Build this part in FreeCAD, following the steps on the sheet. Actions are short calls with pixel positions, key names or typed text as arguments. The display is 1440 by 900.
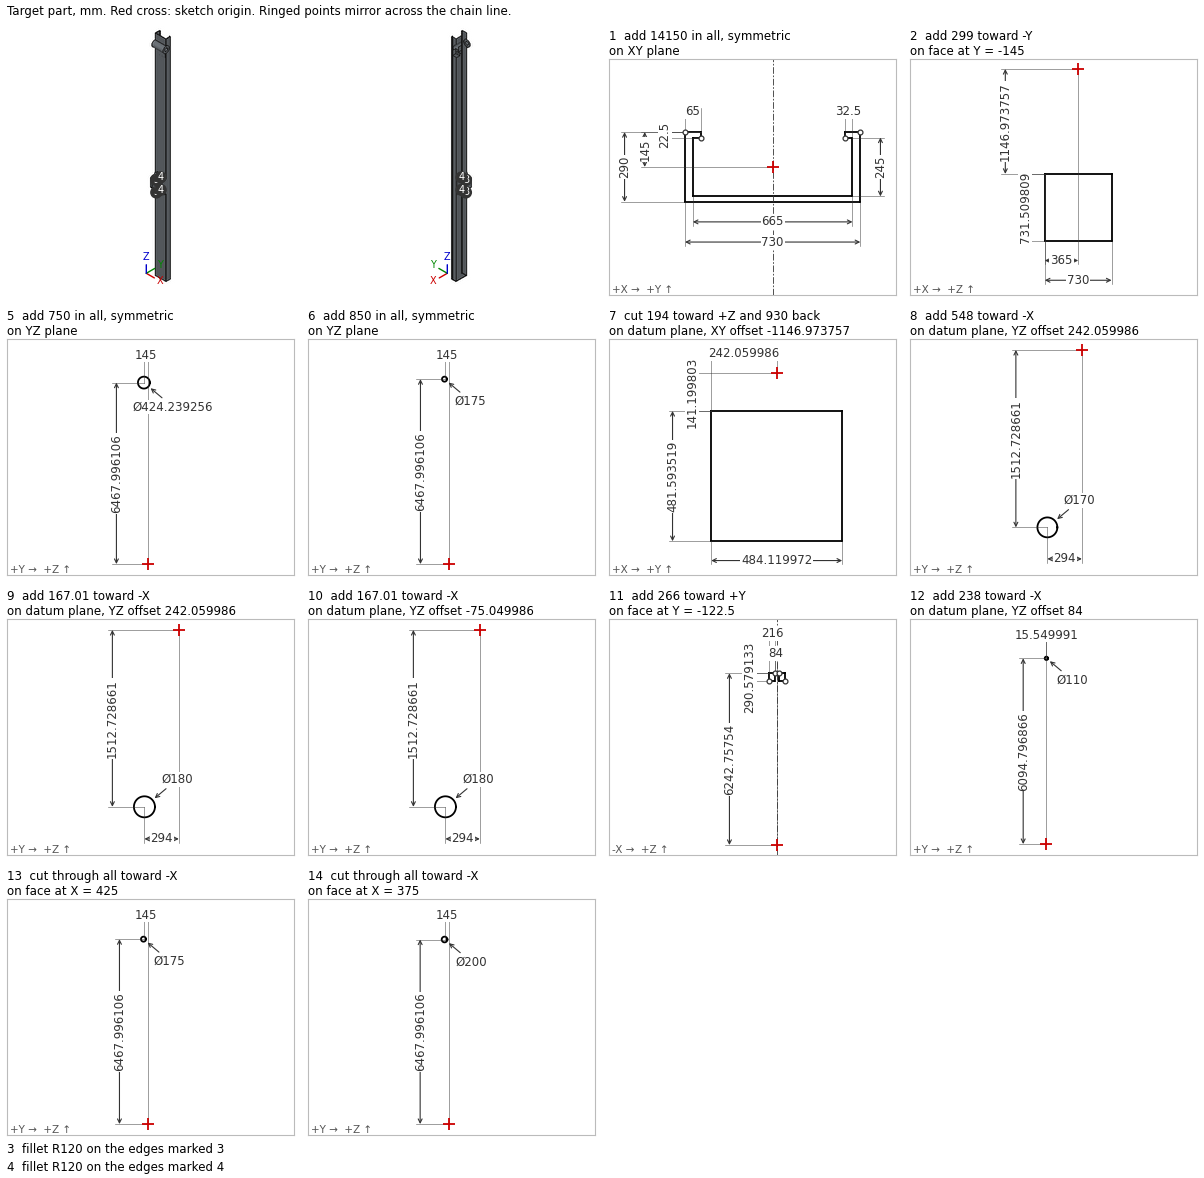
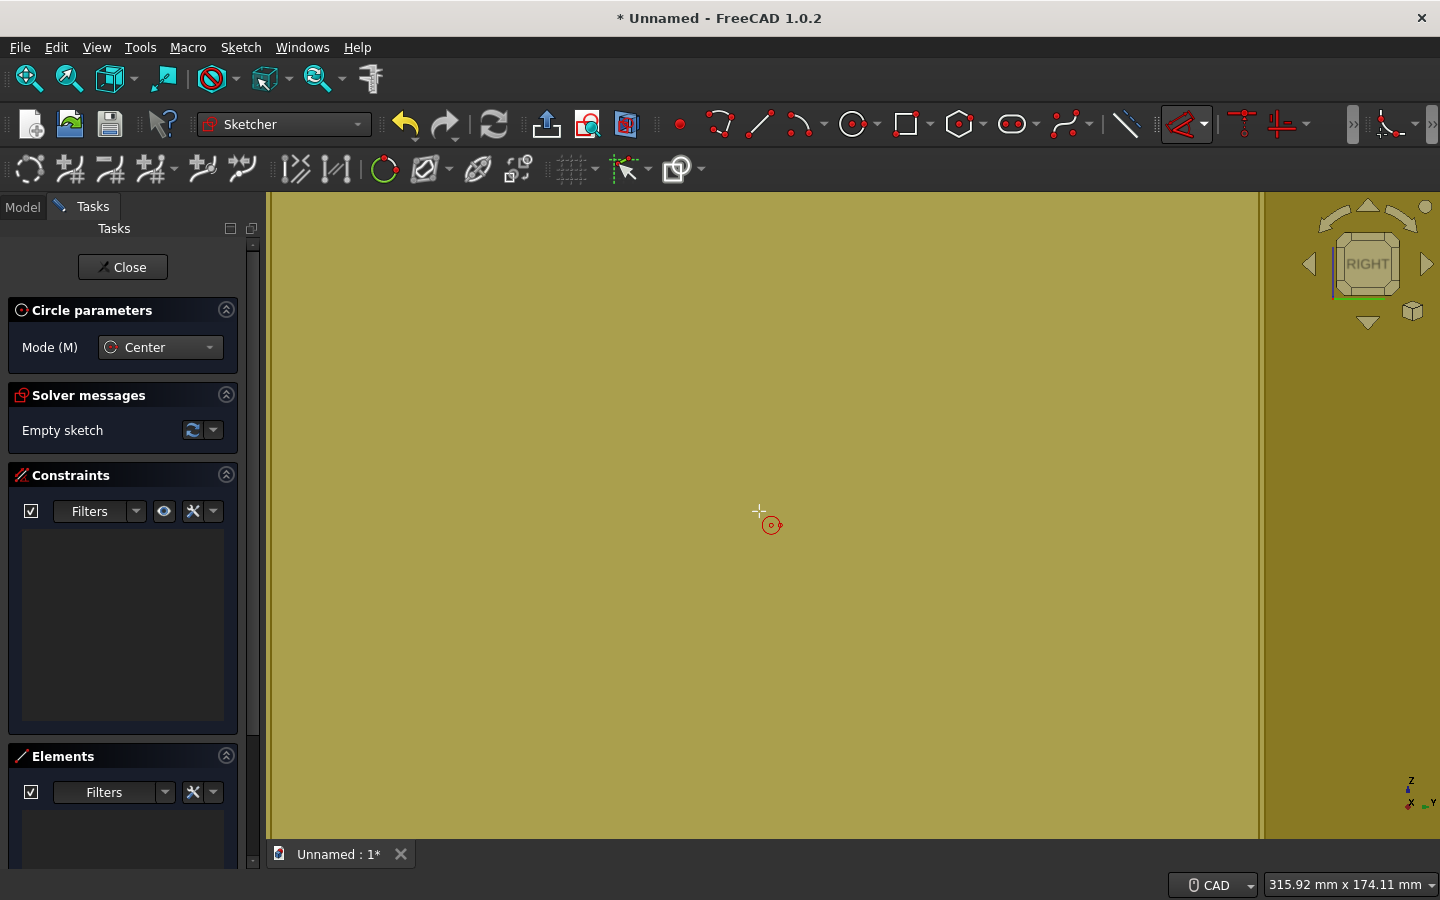
click(784, 513)
click(929, 369)
key(Escape)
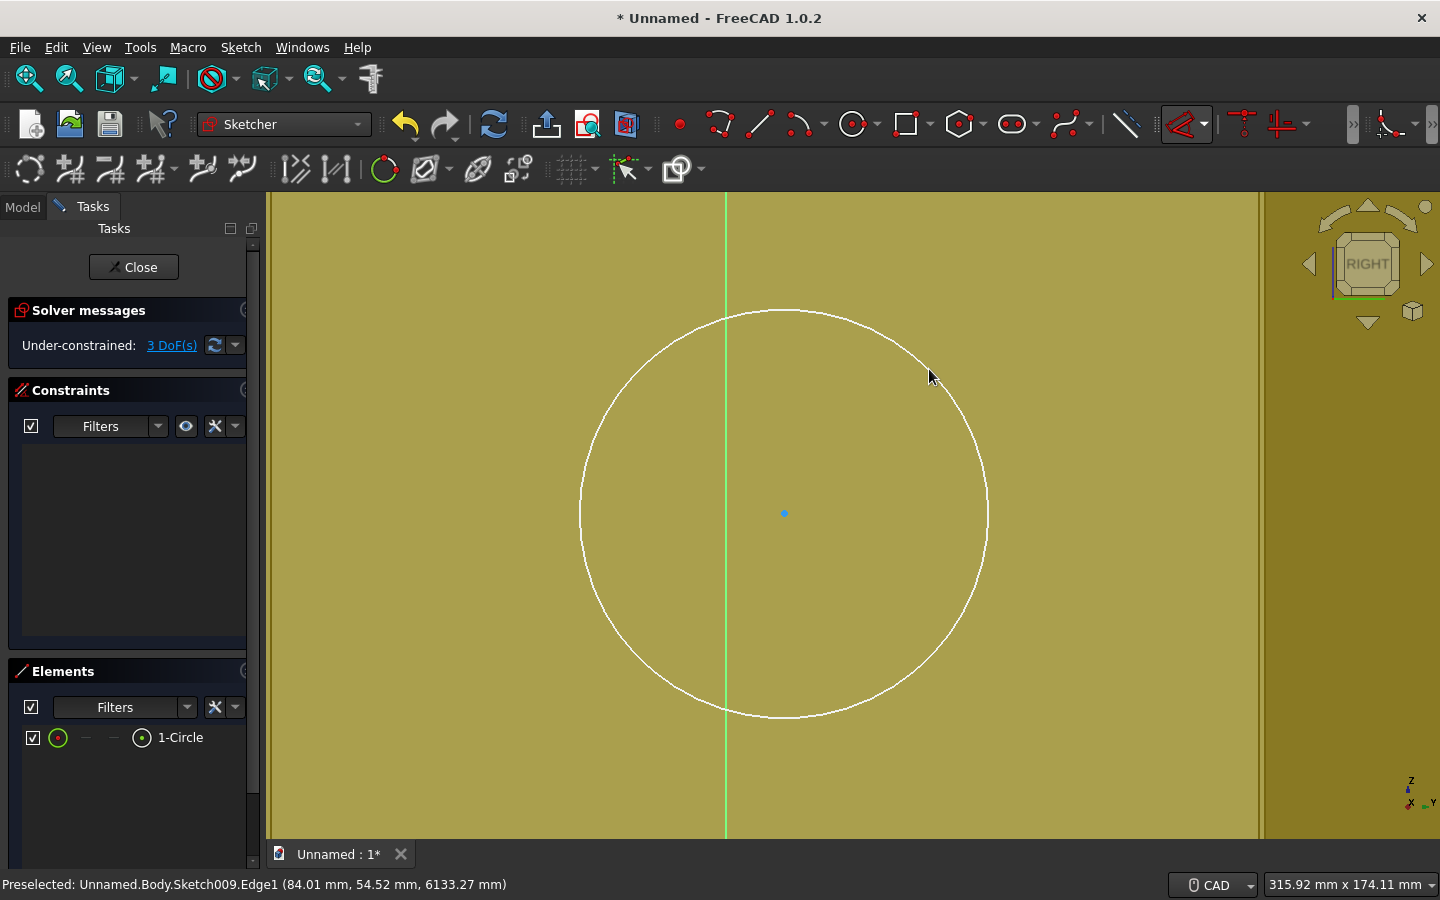
click(928, 369)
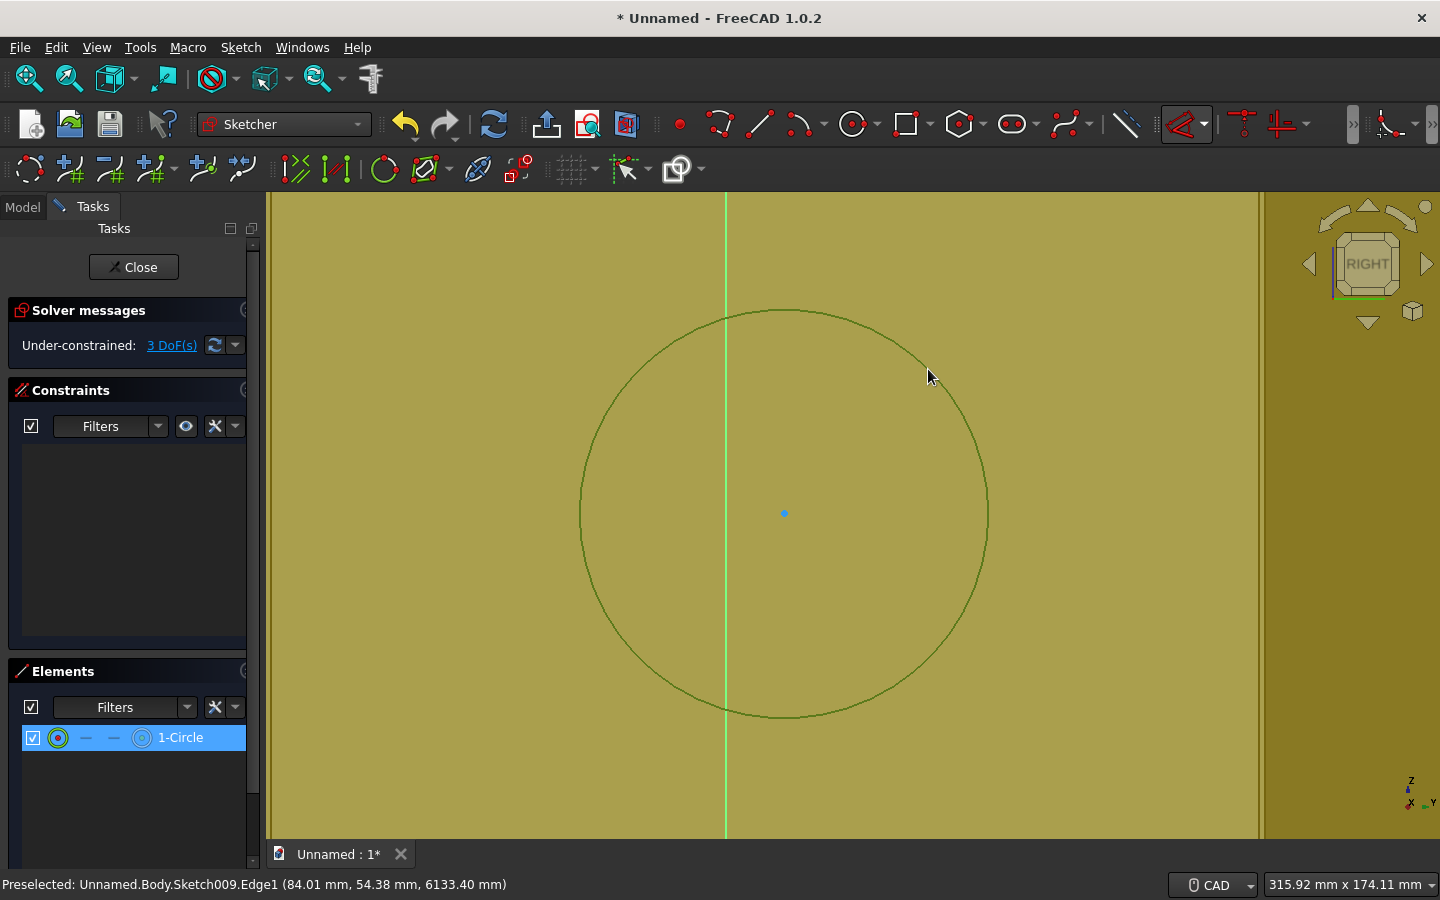
key(k)
key(o)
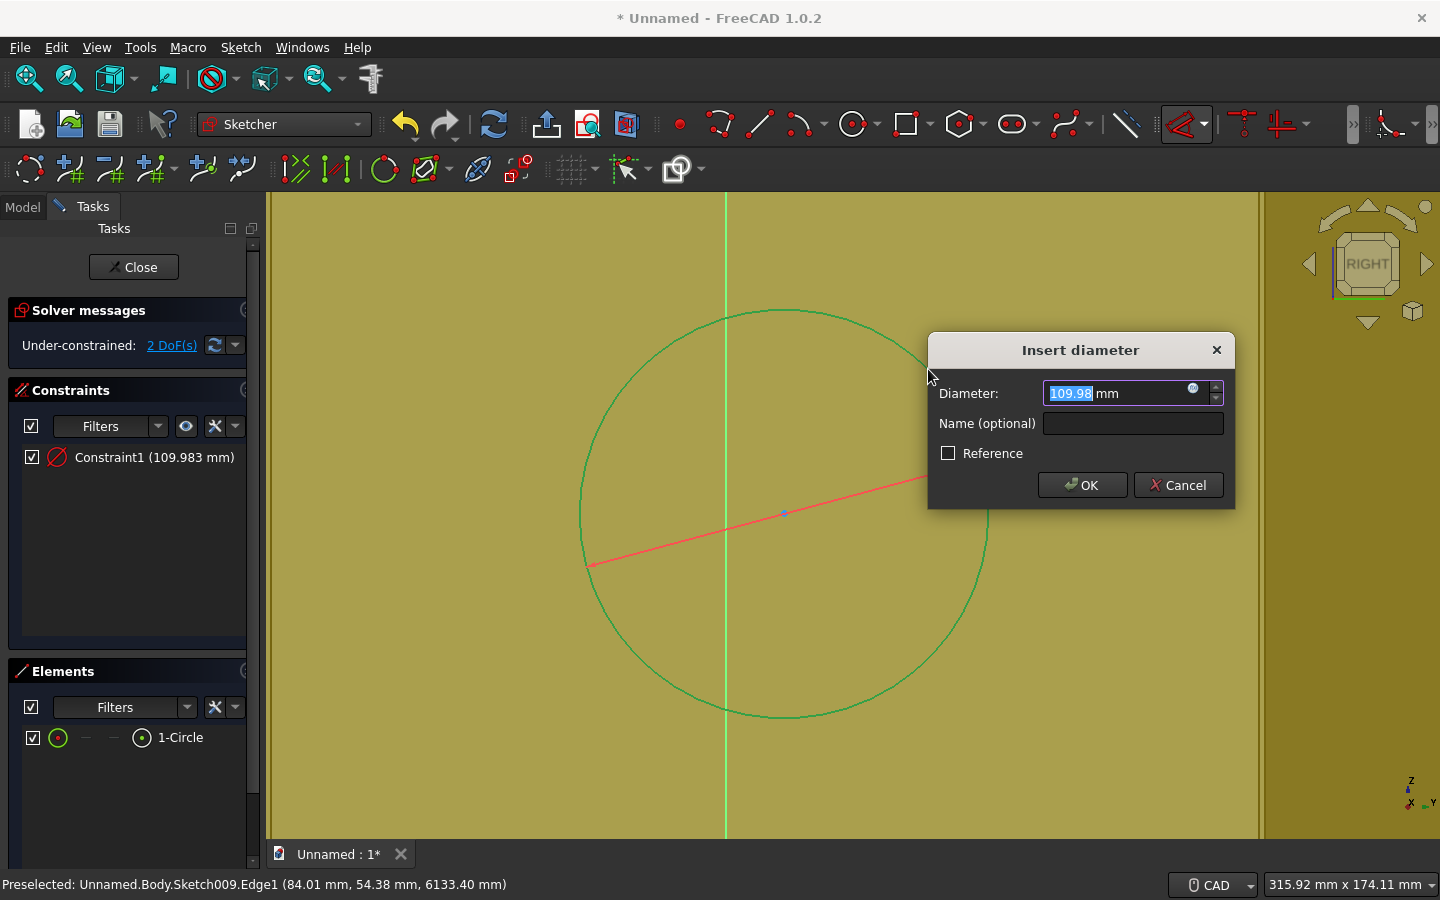
text(110)
key(Return)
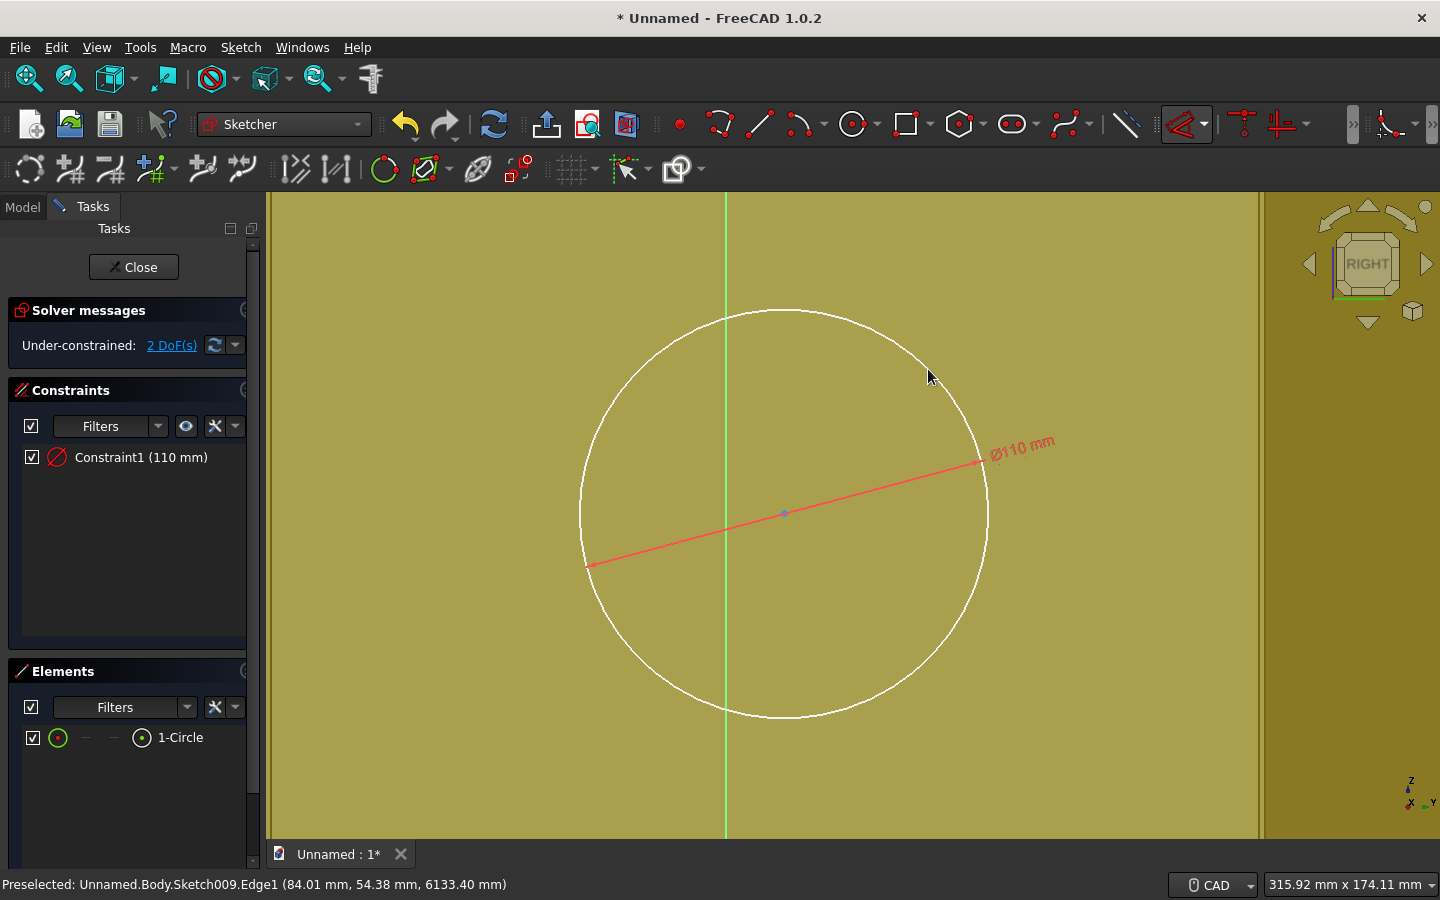
click(784, 514)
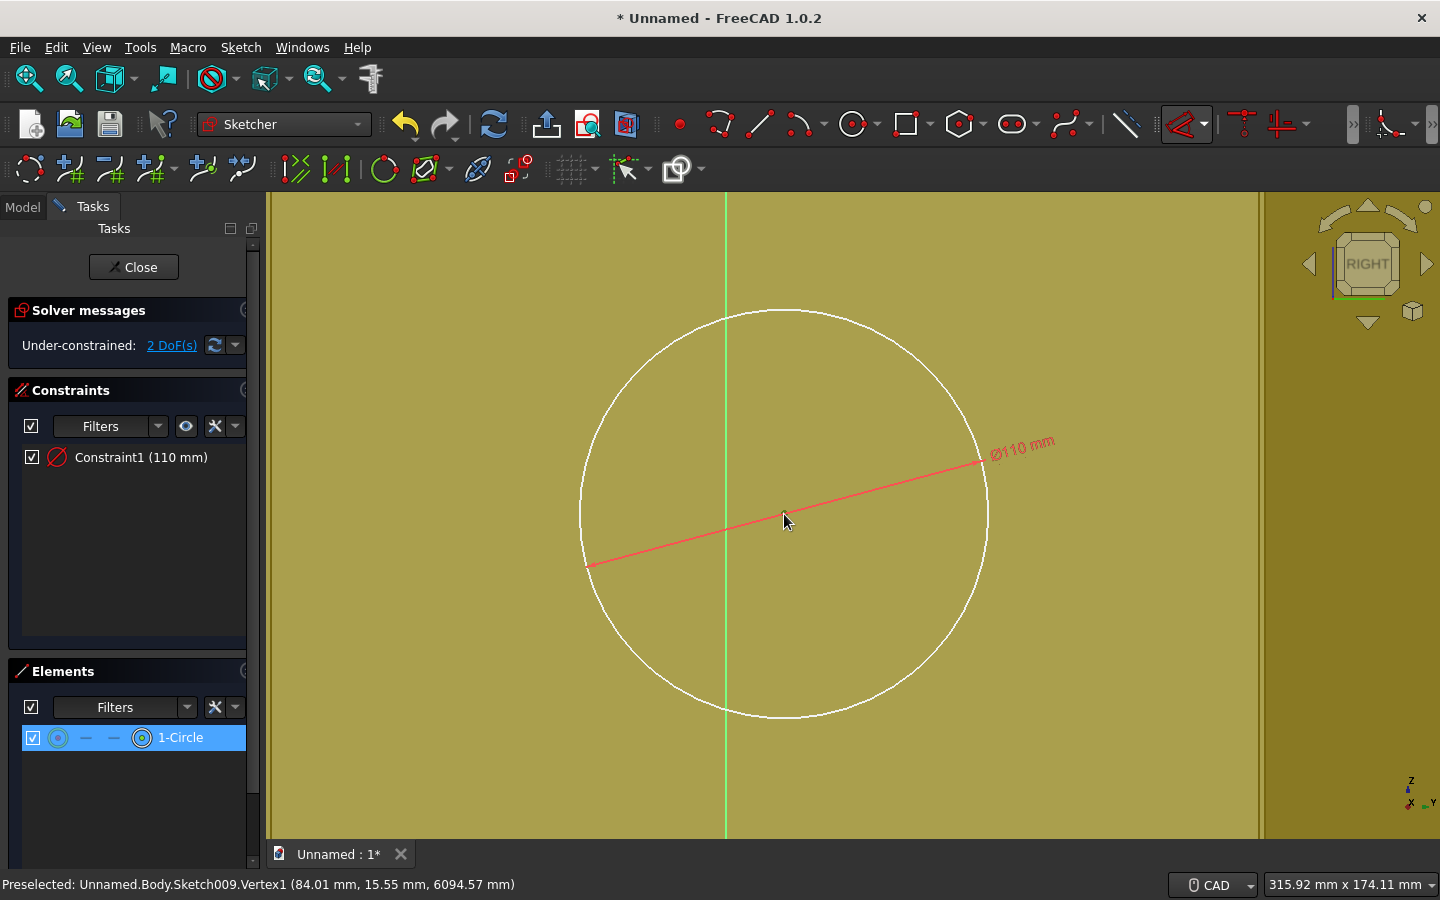
click(1206, 124)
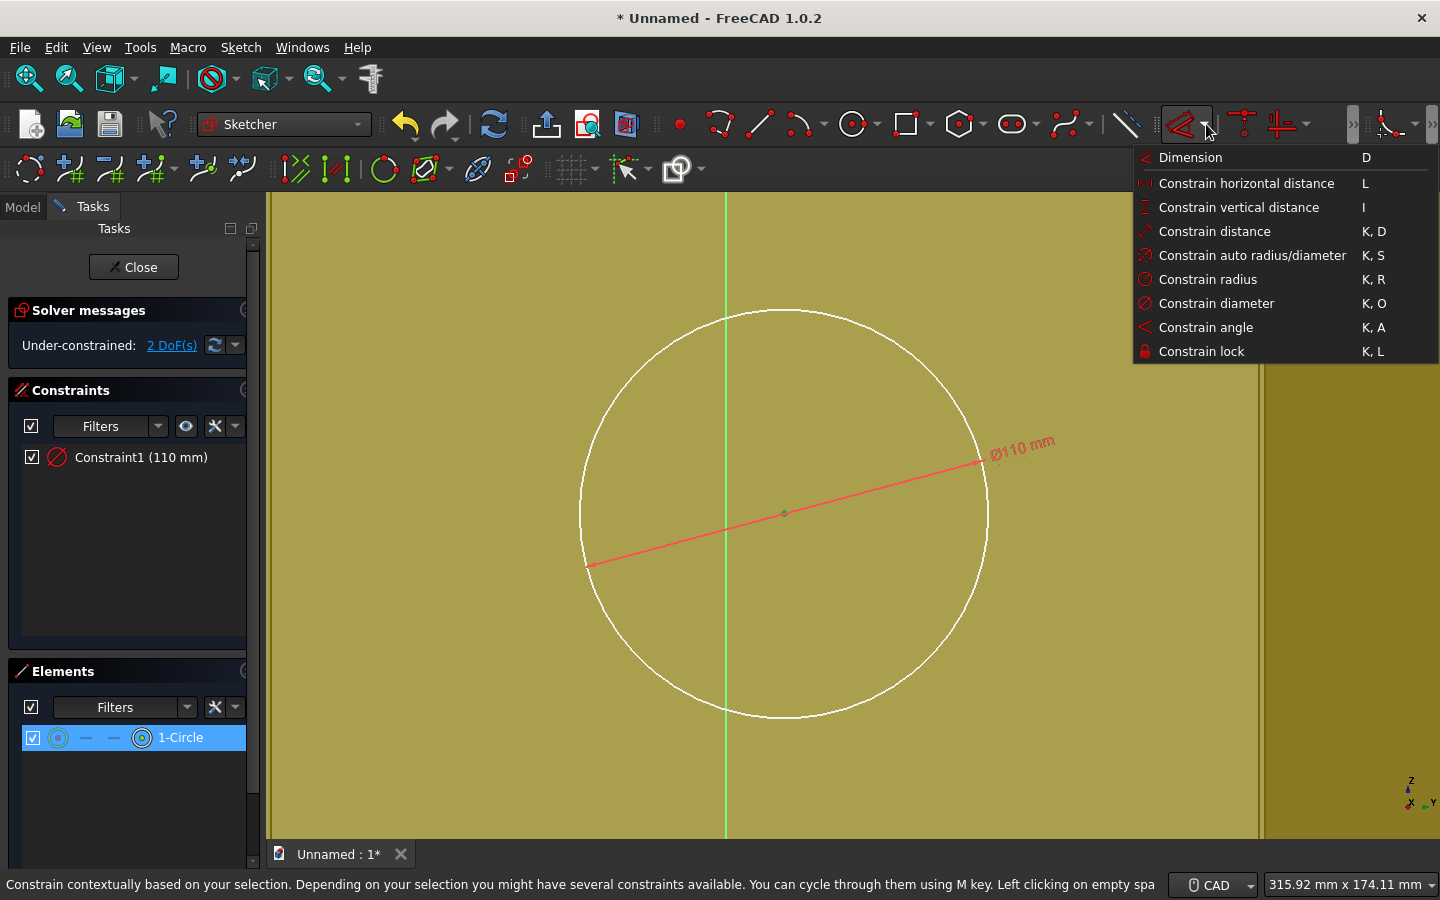
click(1286, 183)